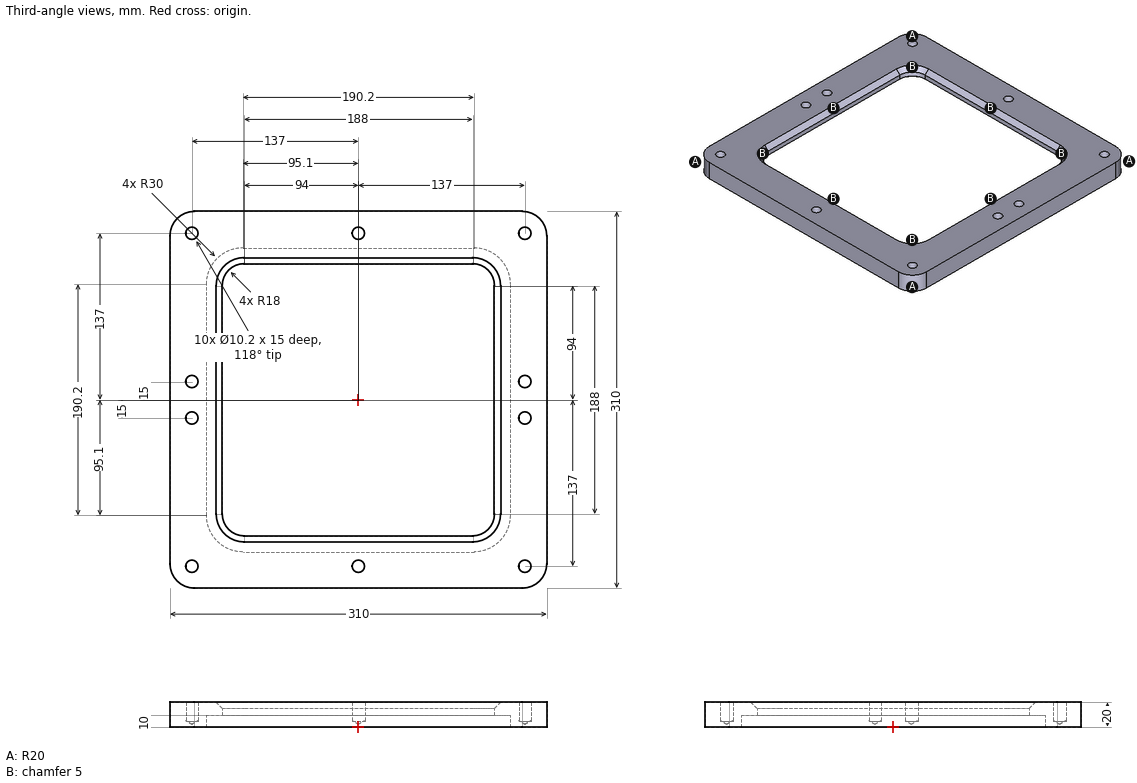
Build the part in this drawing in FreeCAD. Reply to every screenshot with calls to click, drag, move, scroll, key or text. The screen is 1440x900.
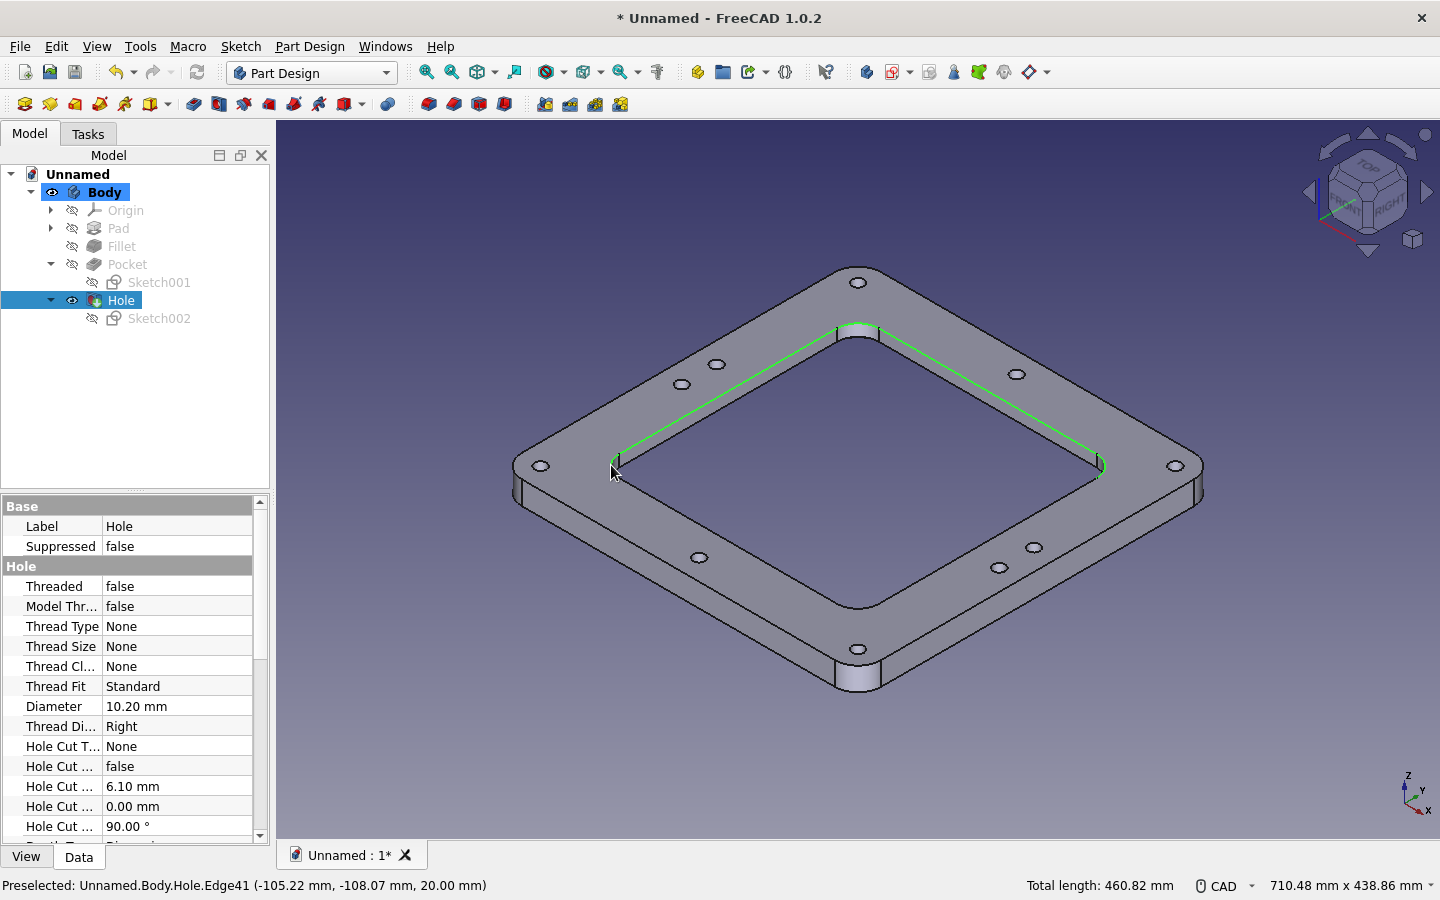
key(2)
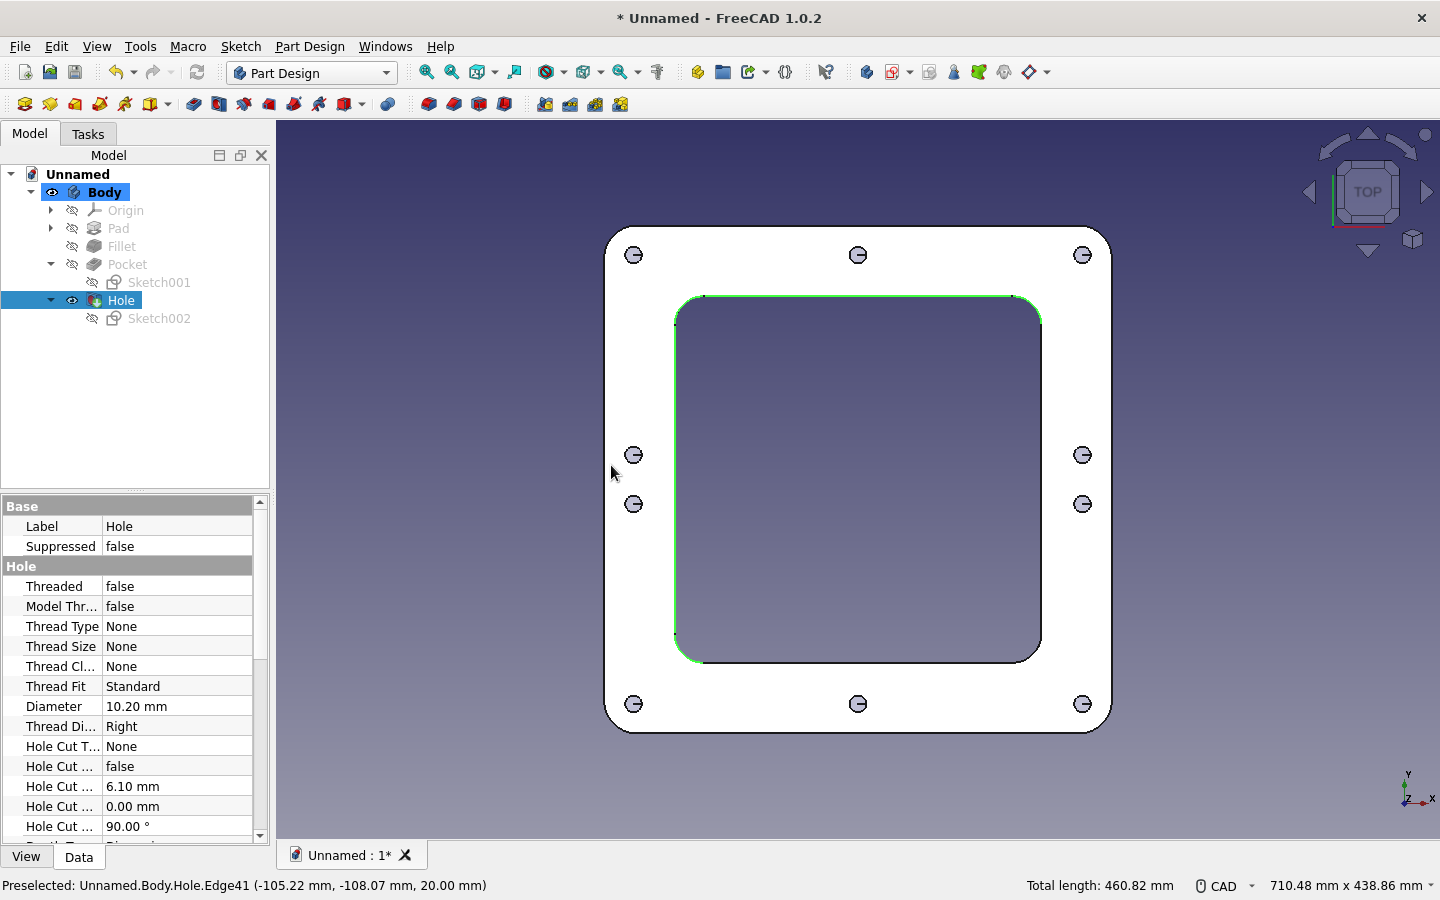
click(1033, 653, ctrl)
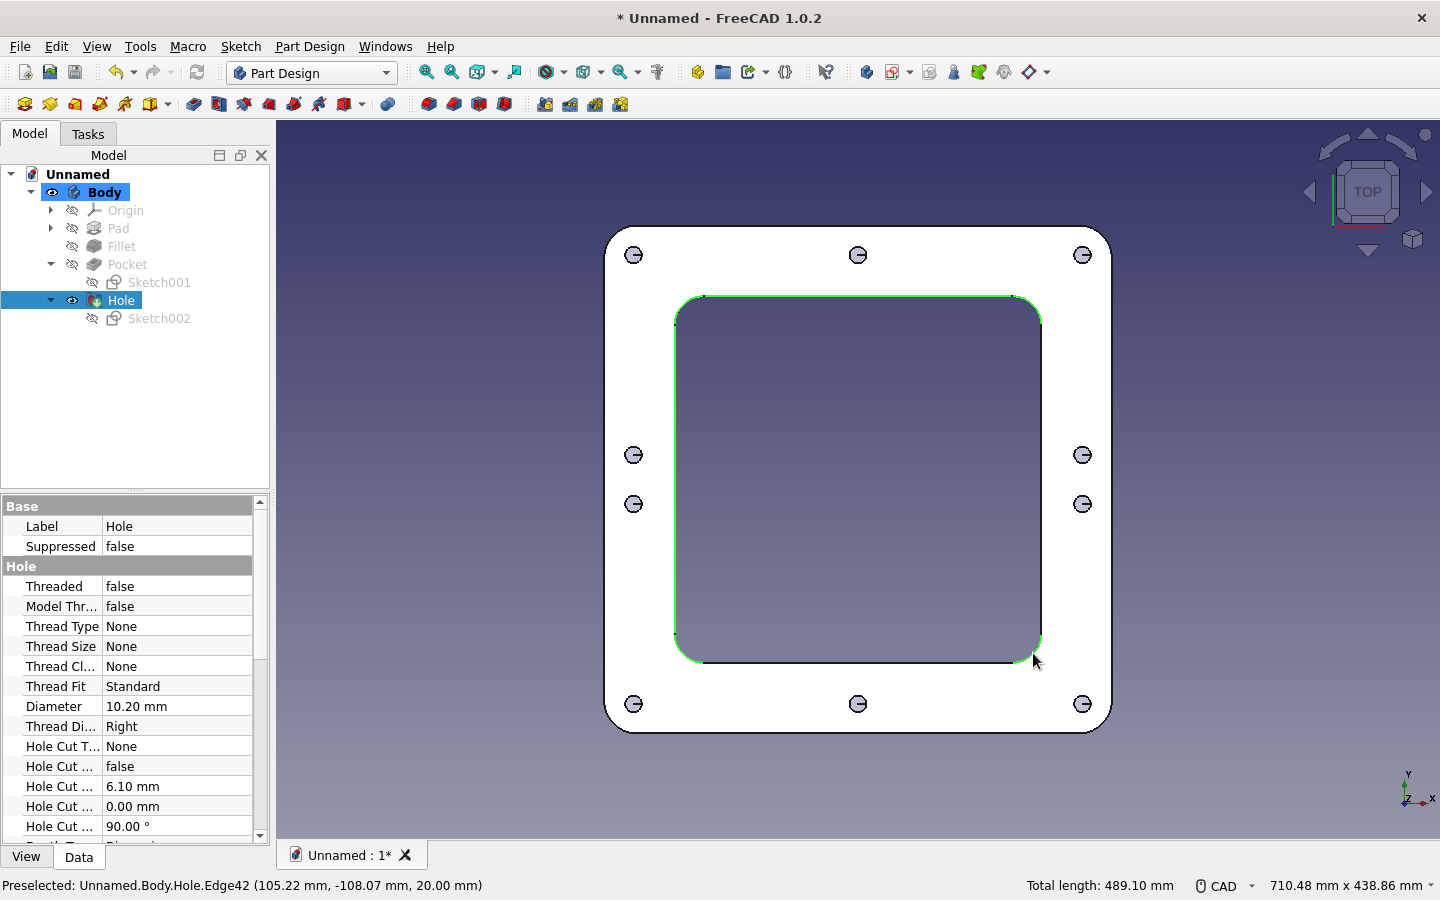
click(1041, 478, ctrl)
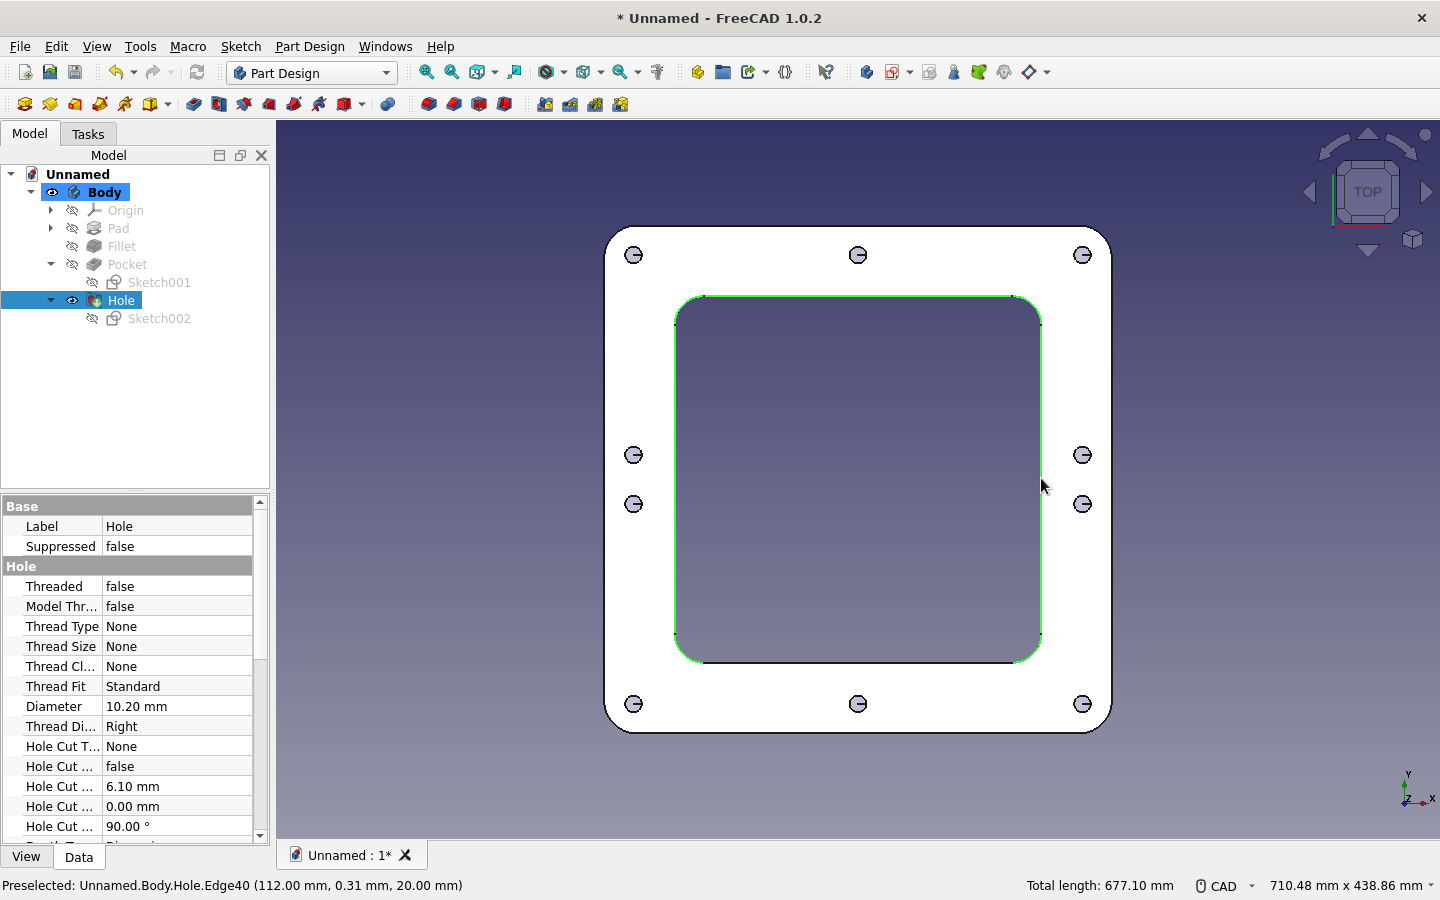
click(858, 662, ctrl)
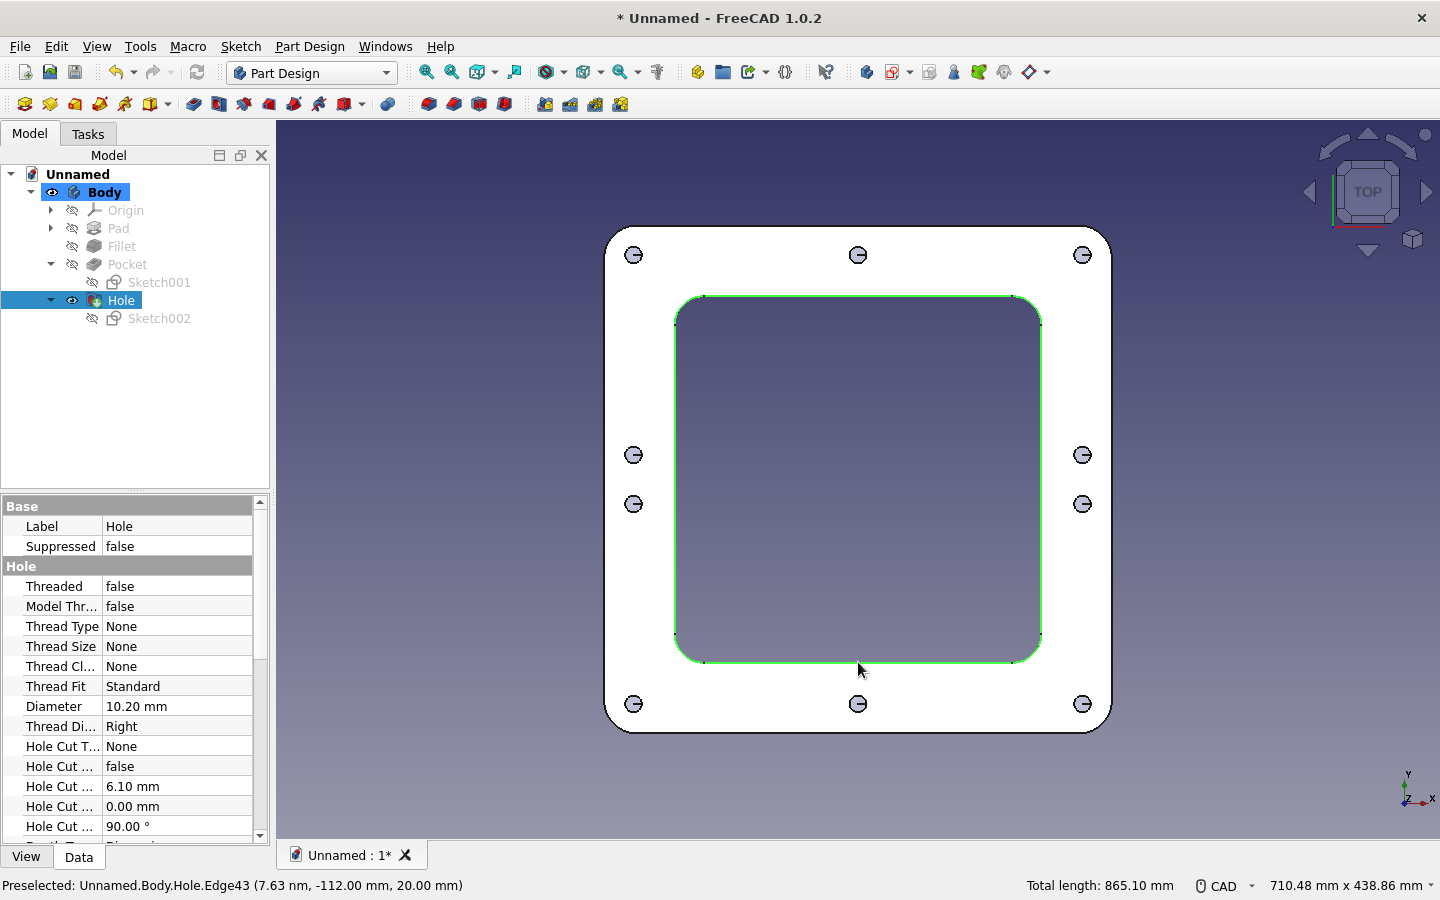
click(454, 104)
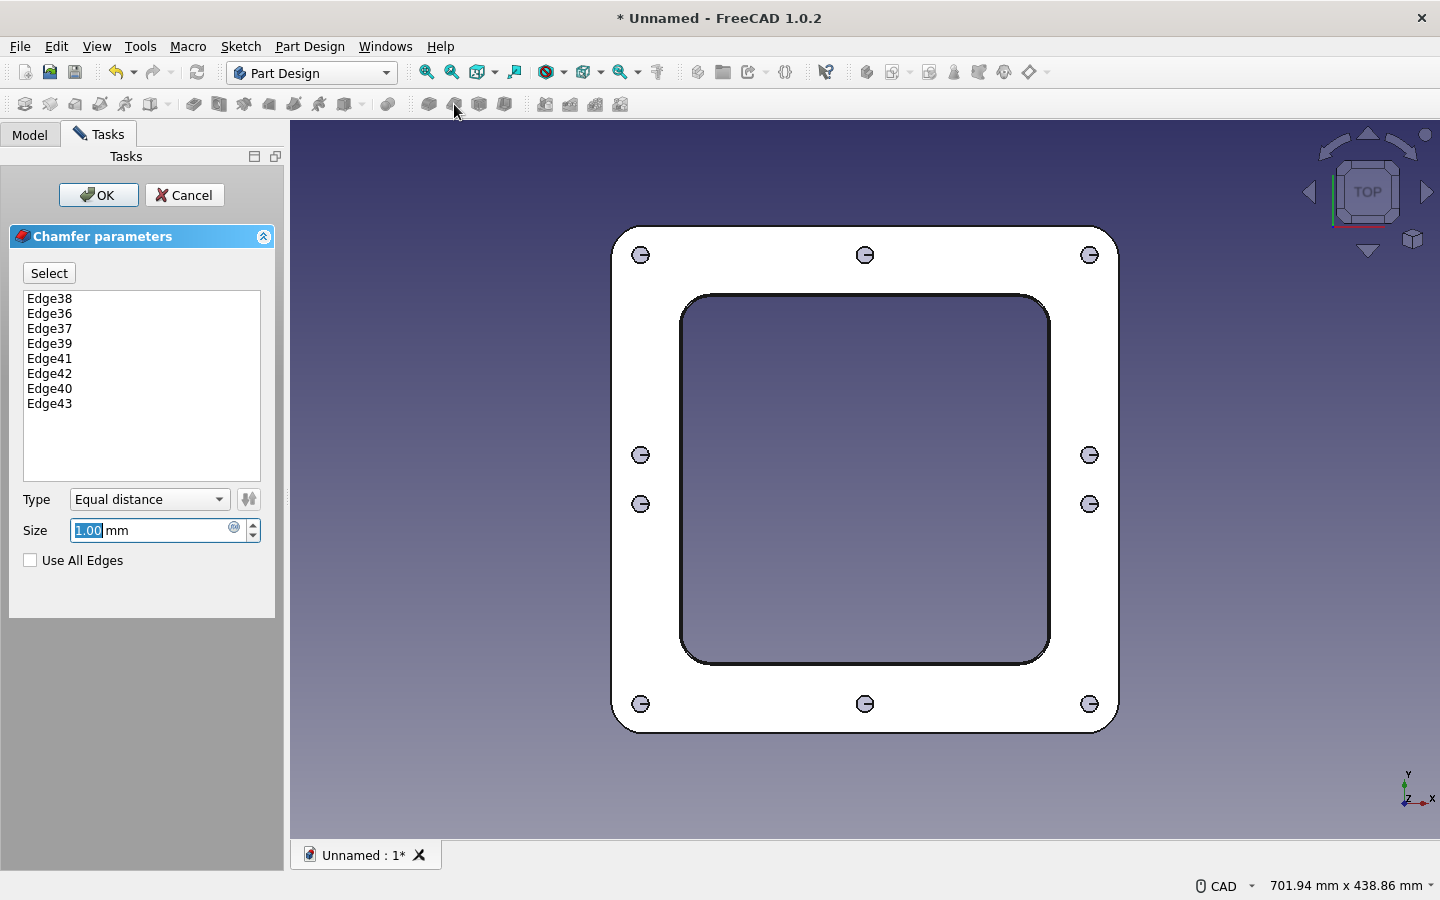
text(5)
key(Tab)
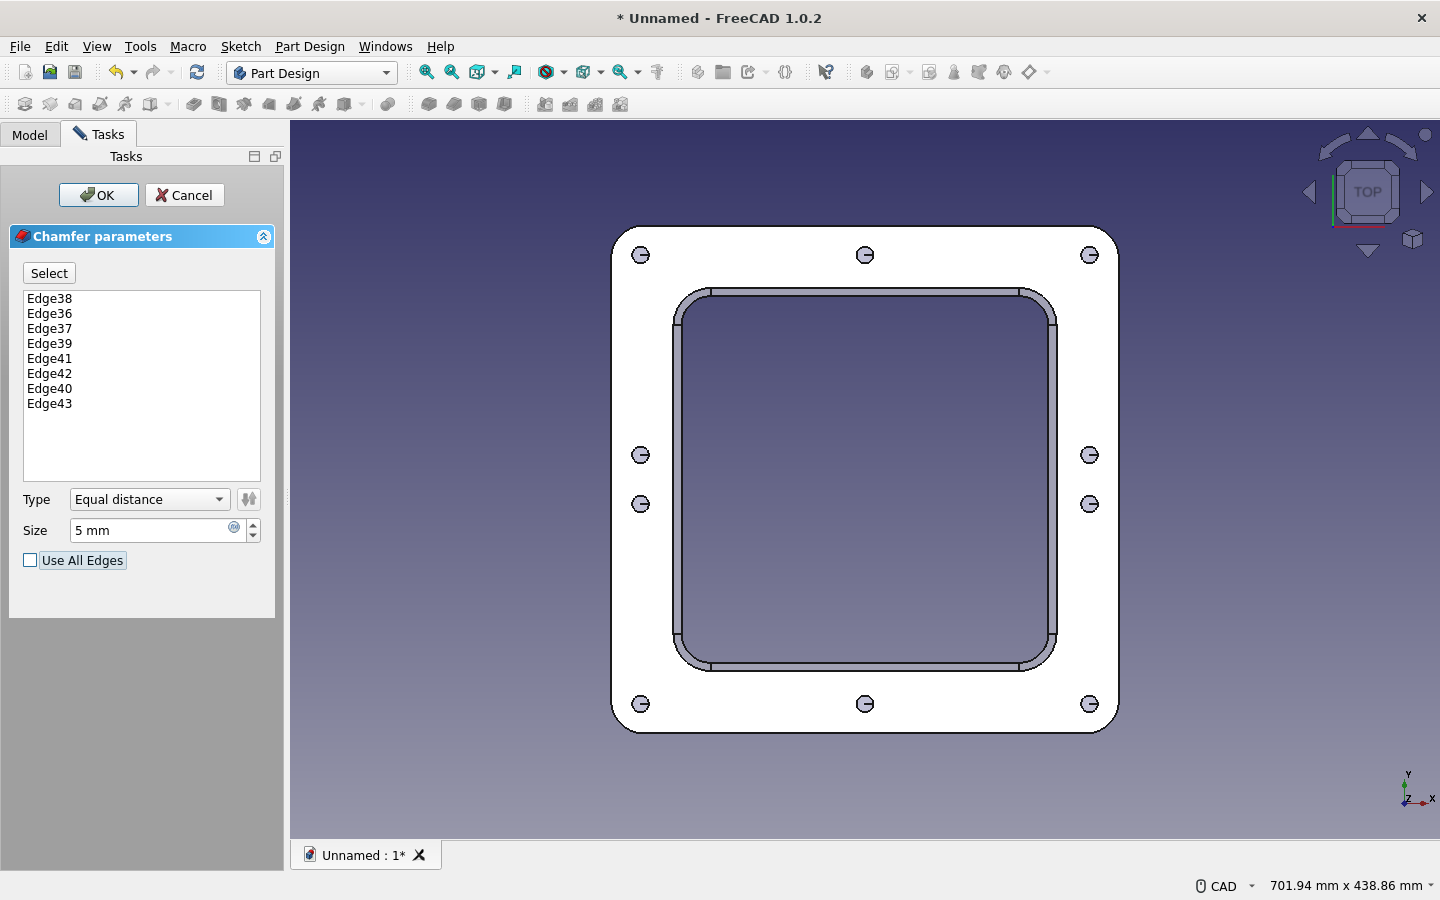
click(99, 195)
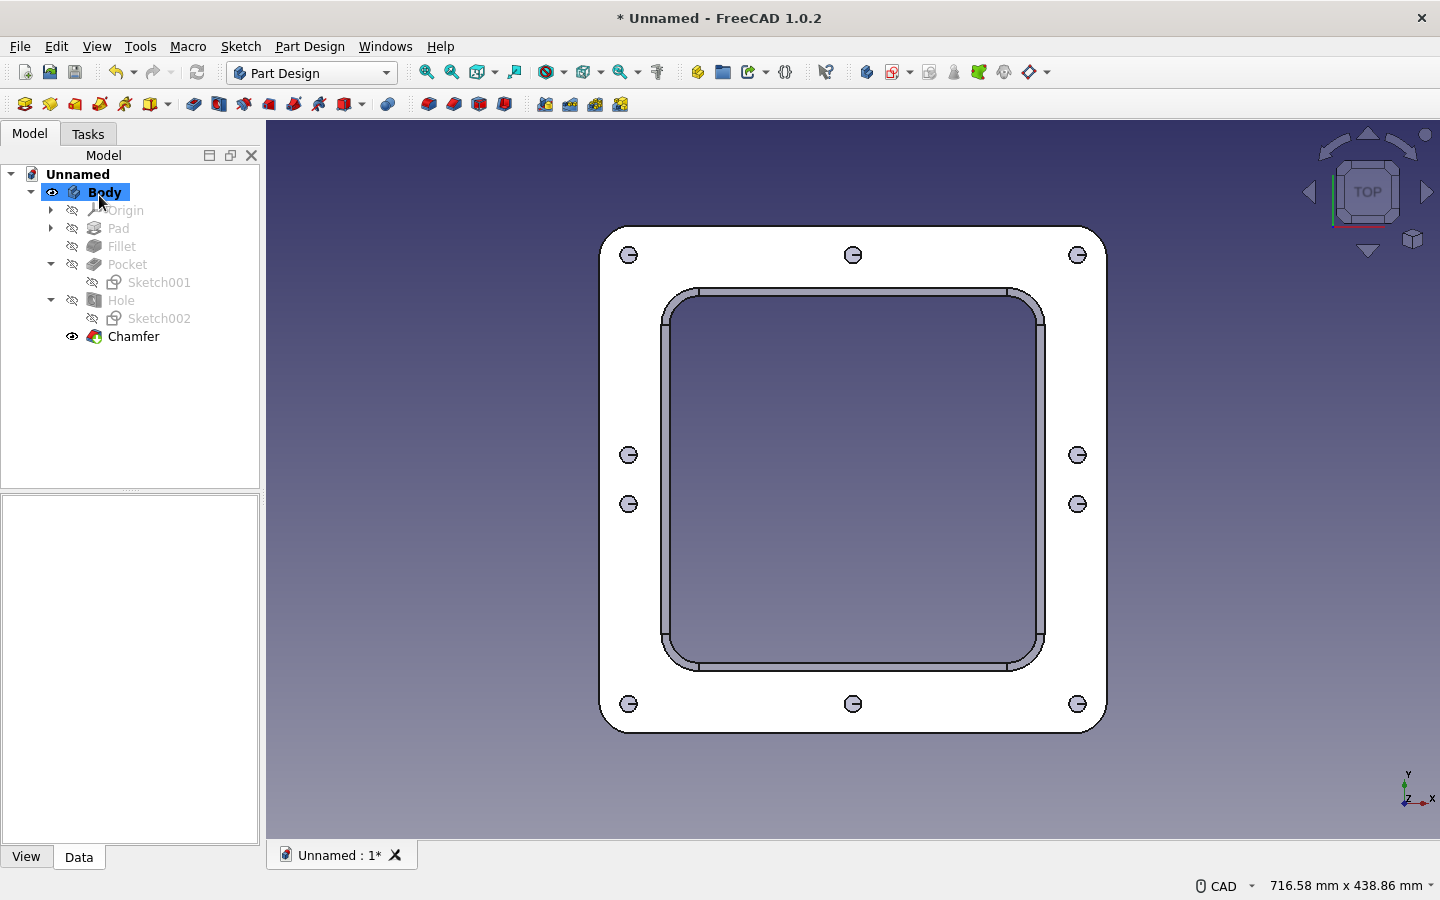
key(0)